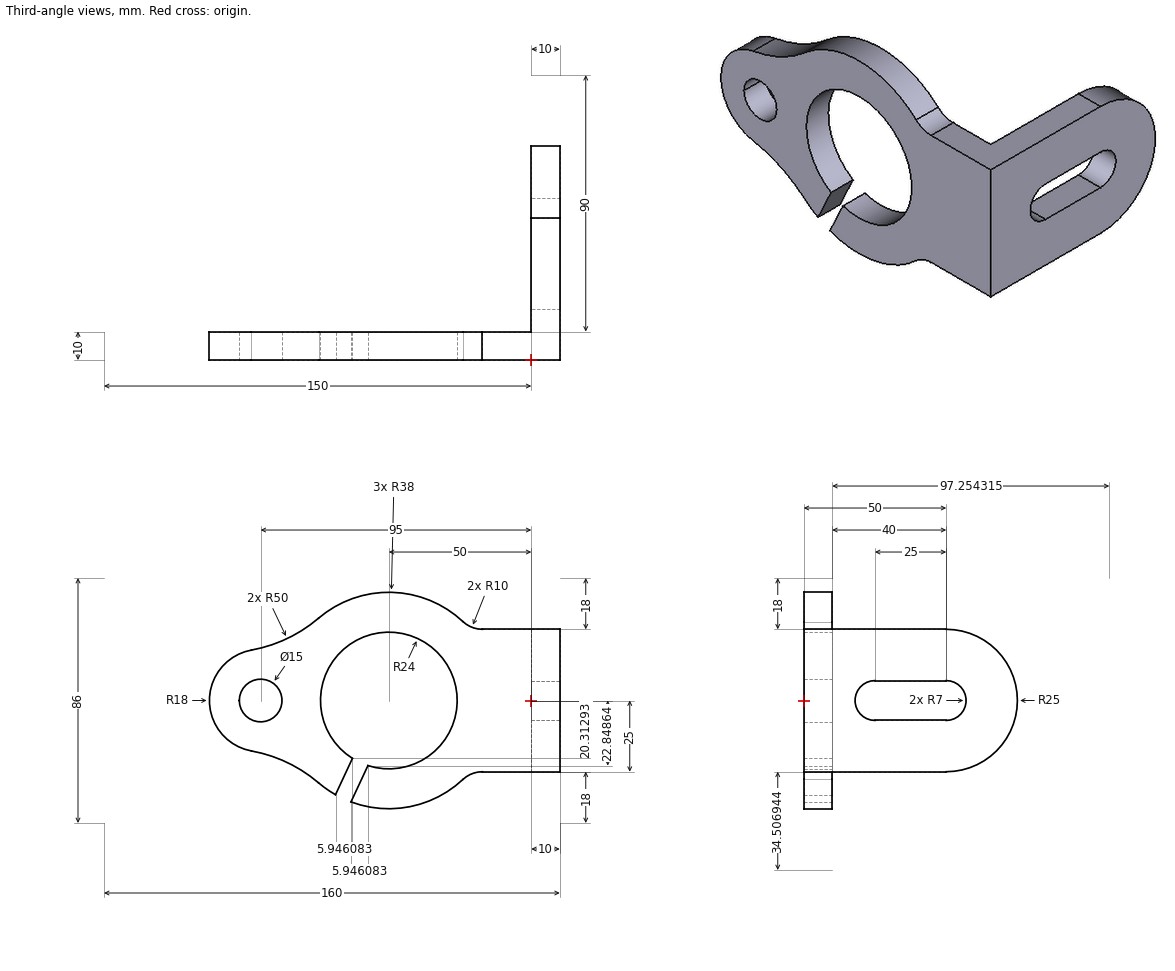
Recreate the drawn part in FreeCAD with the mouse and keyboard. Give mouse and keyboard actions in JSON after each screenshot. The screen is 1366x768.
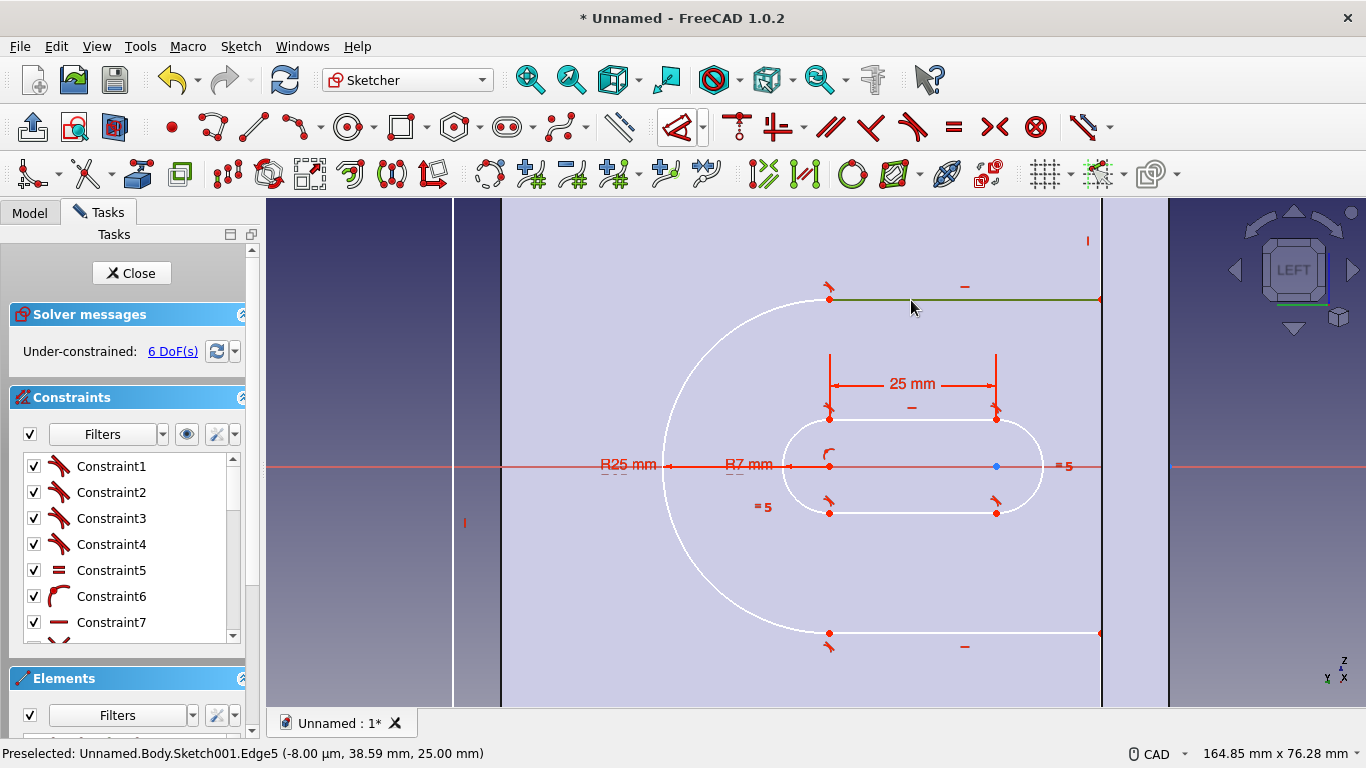
{"action": "key", "text": "l"}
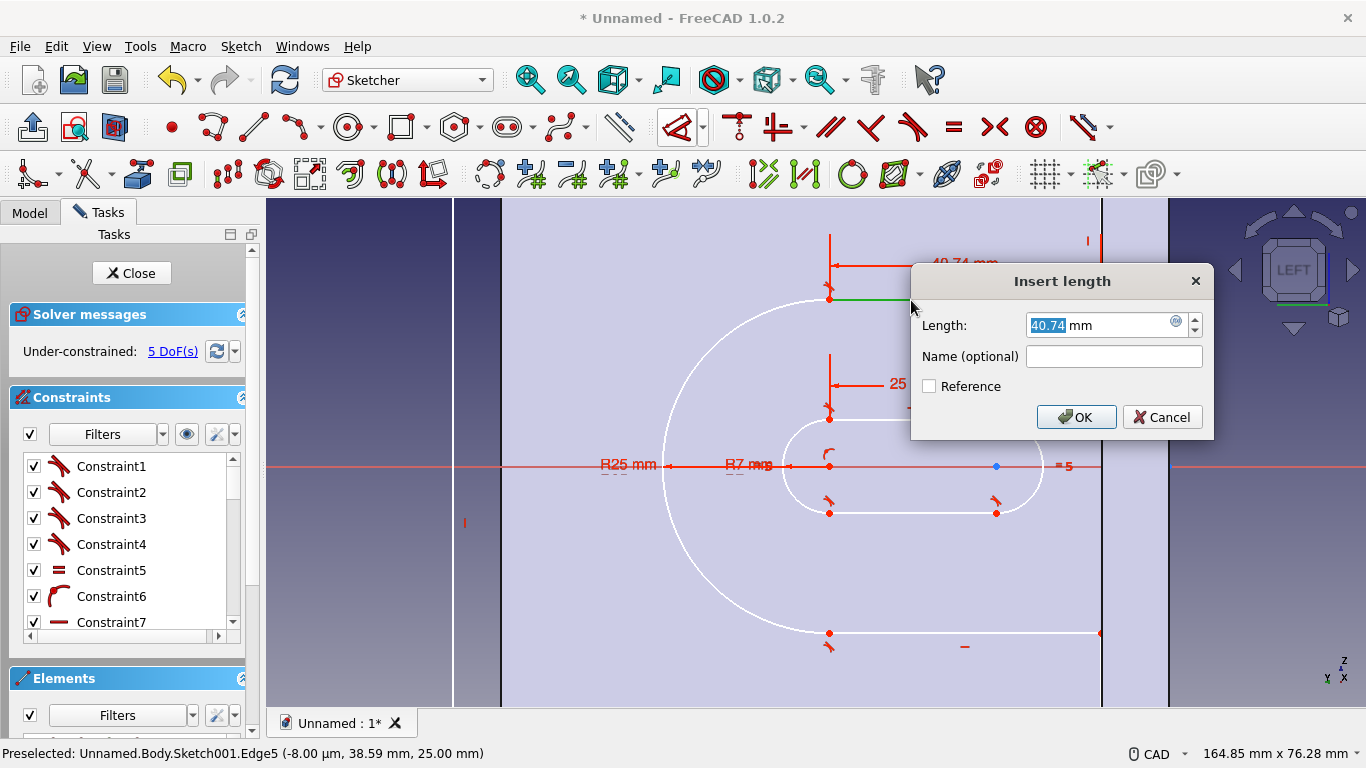
{"action": "type", "text": "40"}
{"action": "key", "text": "Return"}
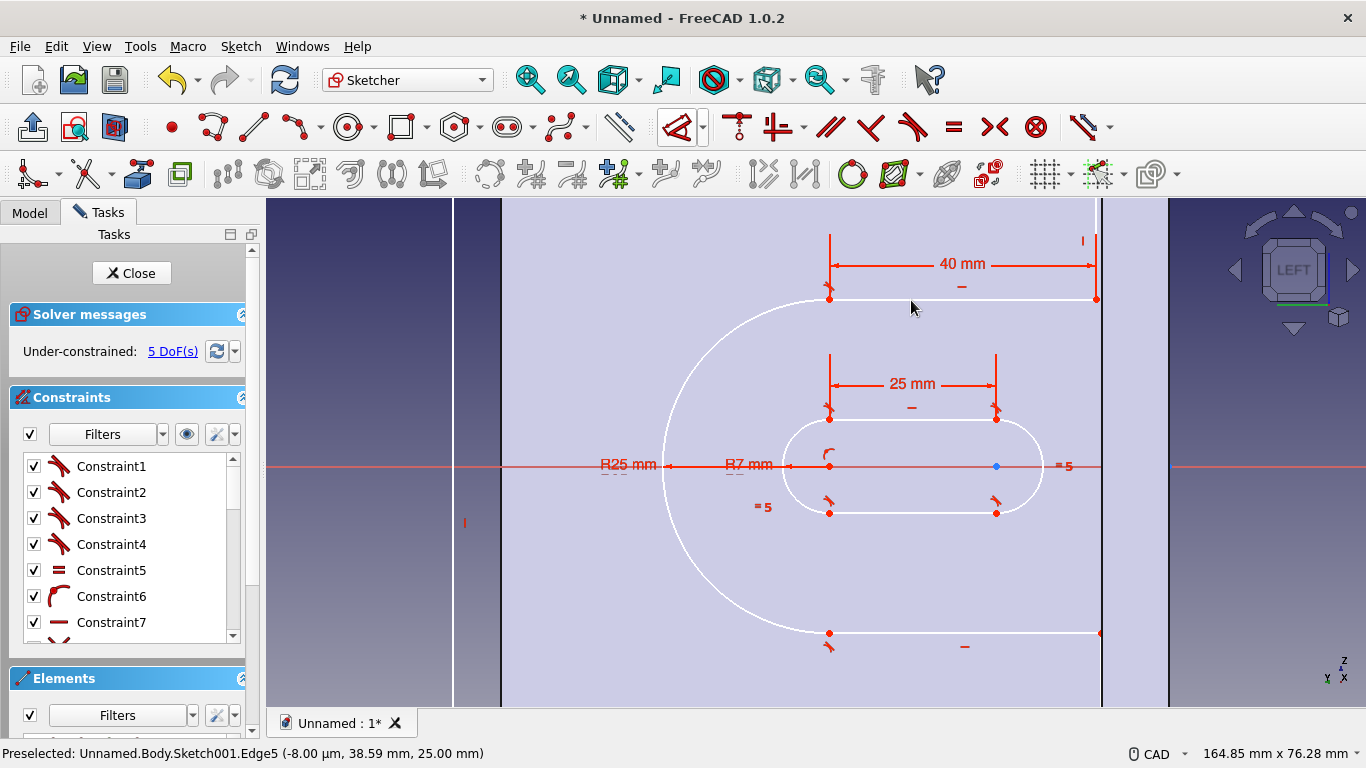
{"action": "left_click", "coordinate": [1096, 264]}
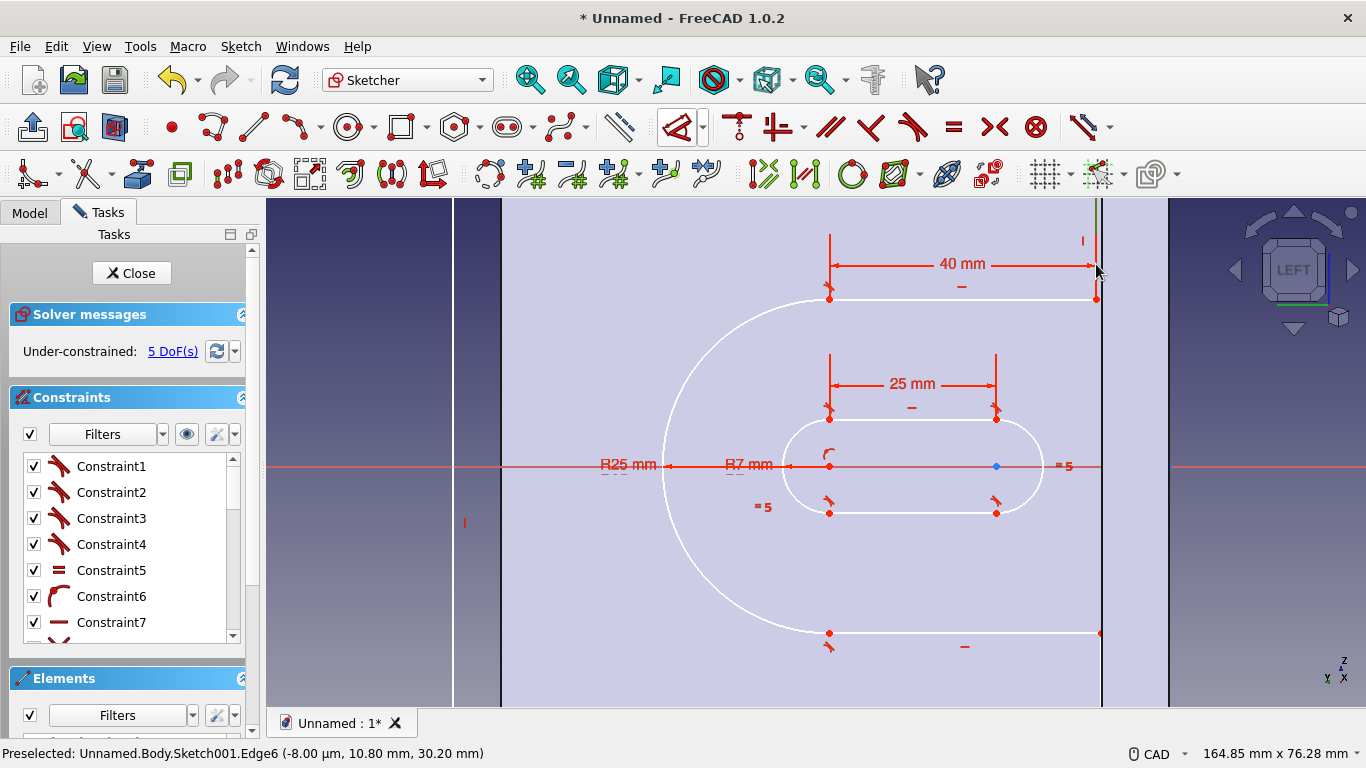
{"action": "key", "text": "i"}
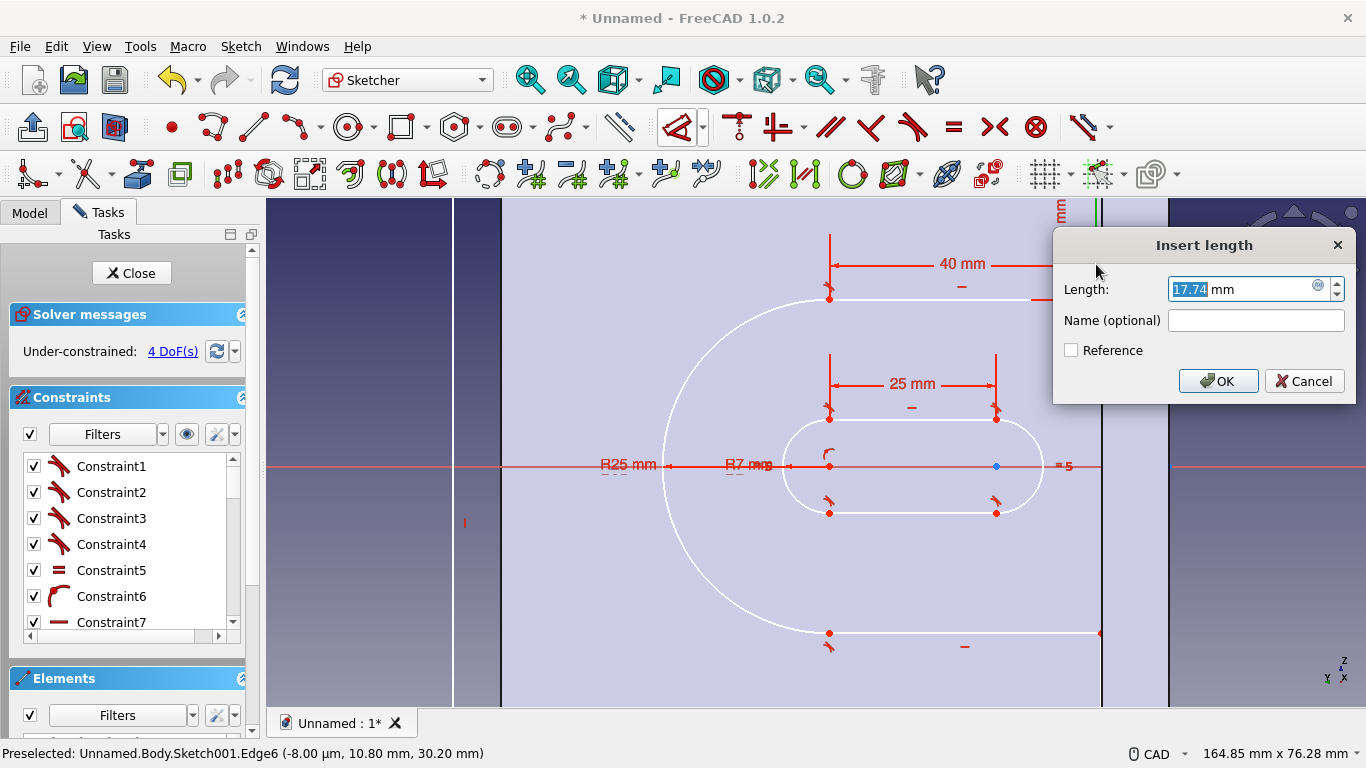
{"action": "type", "text": "18"}
{"action": "key", "text": "Return"}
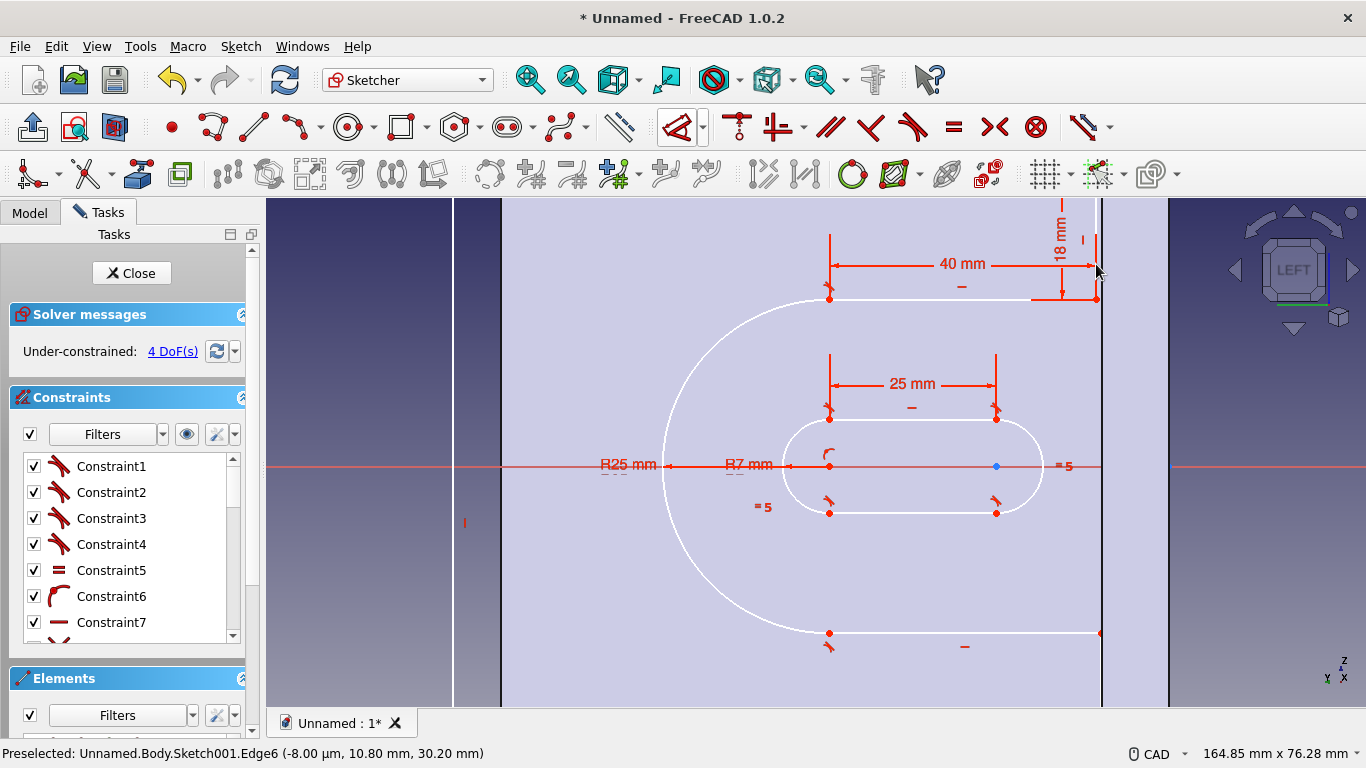
{"action": "left_click", "coordinate": [1020, 633]}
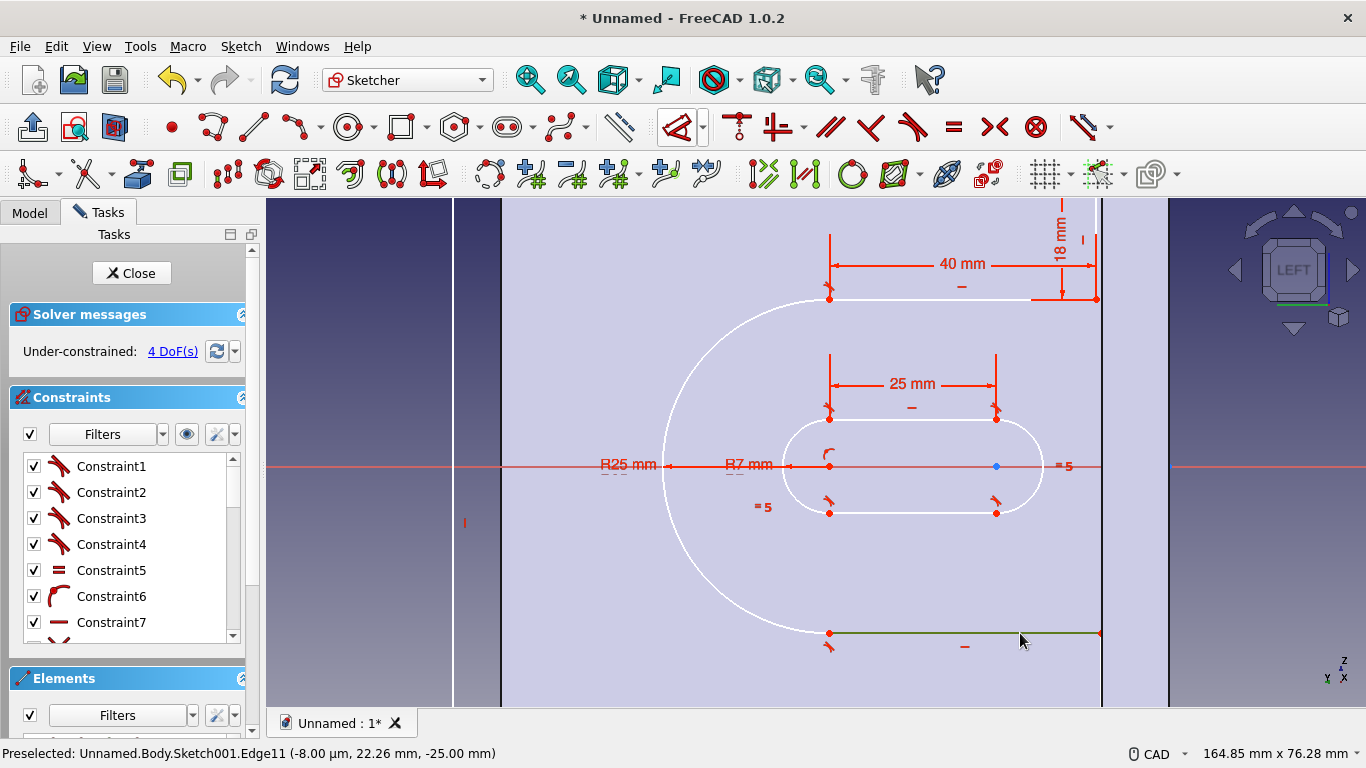
{"action": "key", "text": "l"}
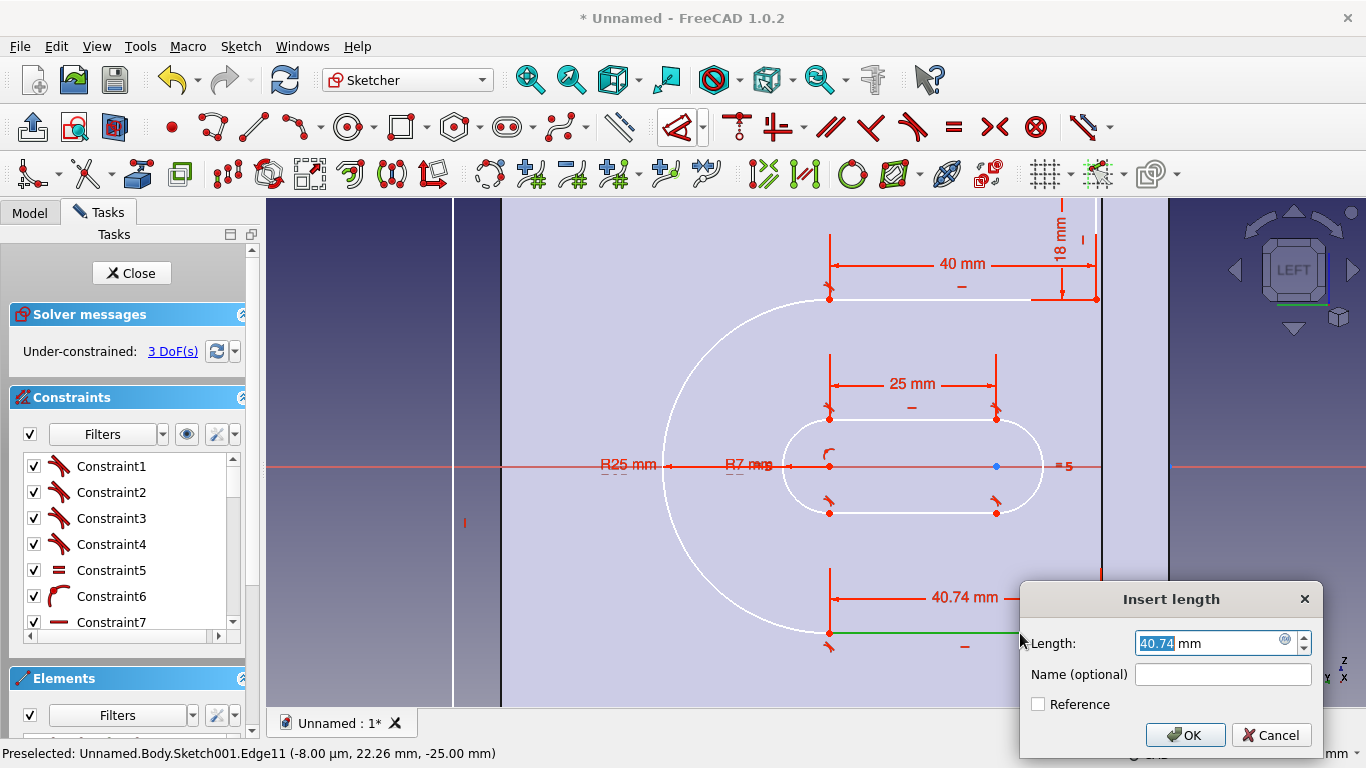
{"action": "type", "text": "40"}
{"action": "key", "text": "Return"}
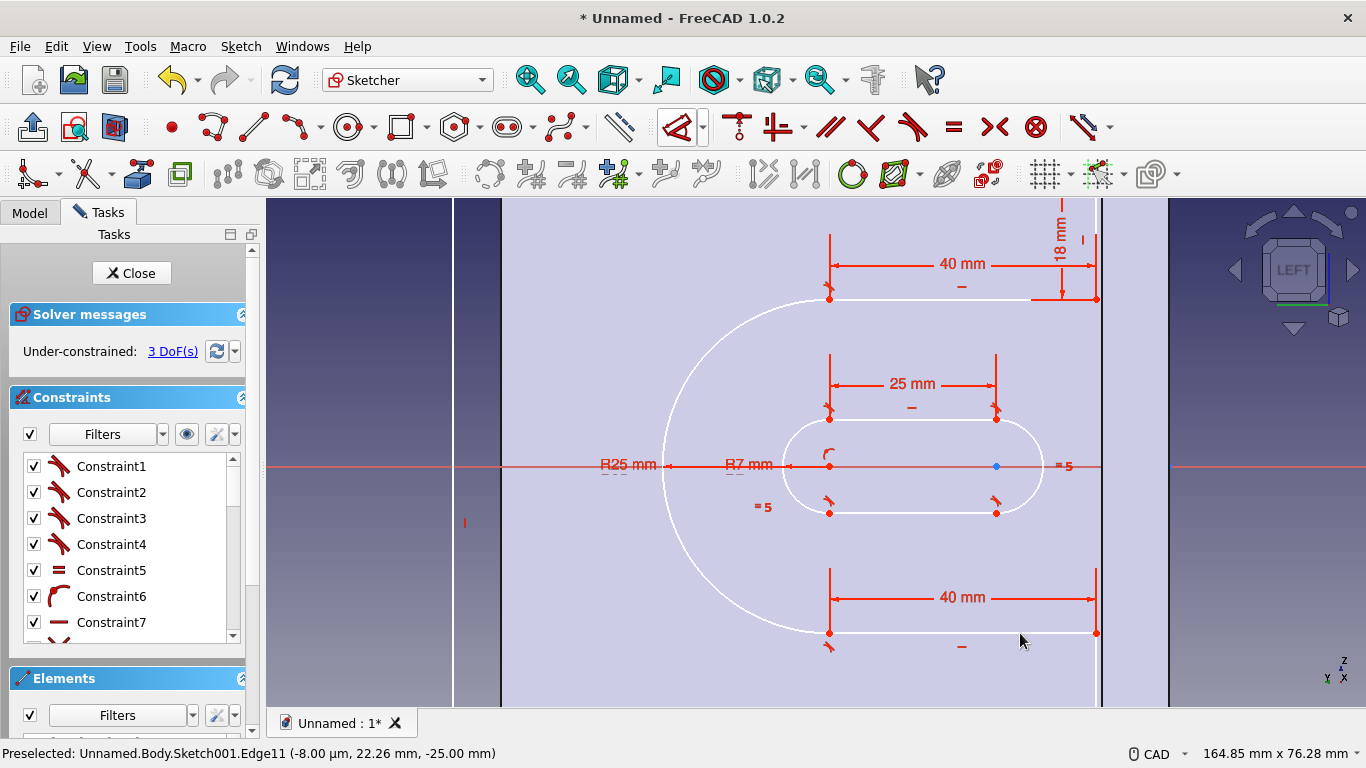
{"action": "left_click", "coordinate": [830, 420]}